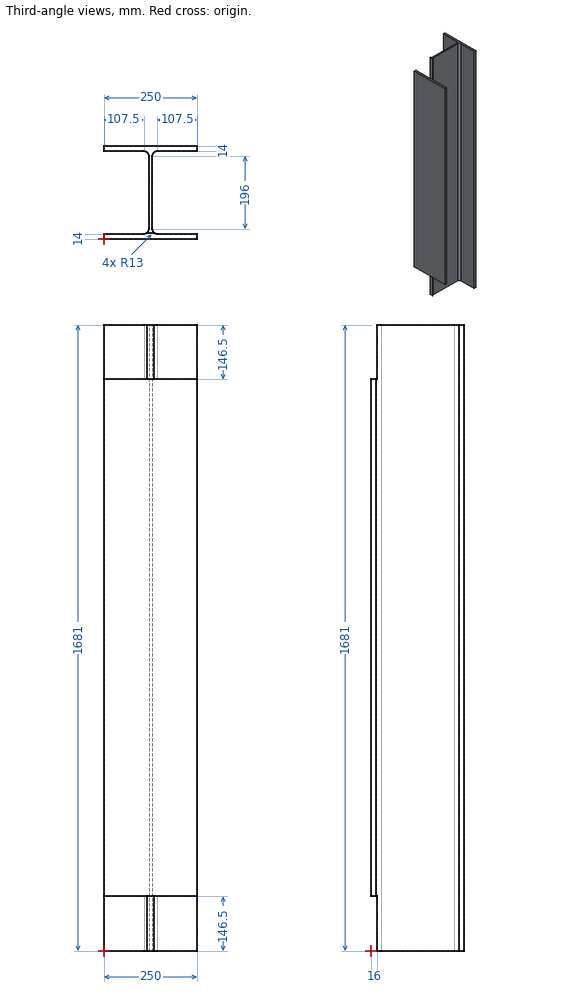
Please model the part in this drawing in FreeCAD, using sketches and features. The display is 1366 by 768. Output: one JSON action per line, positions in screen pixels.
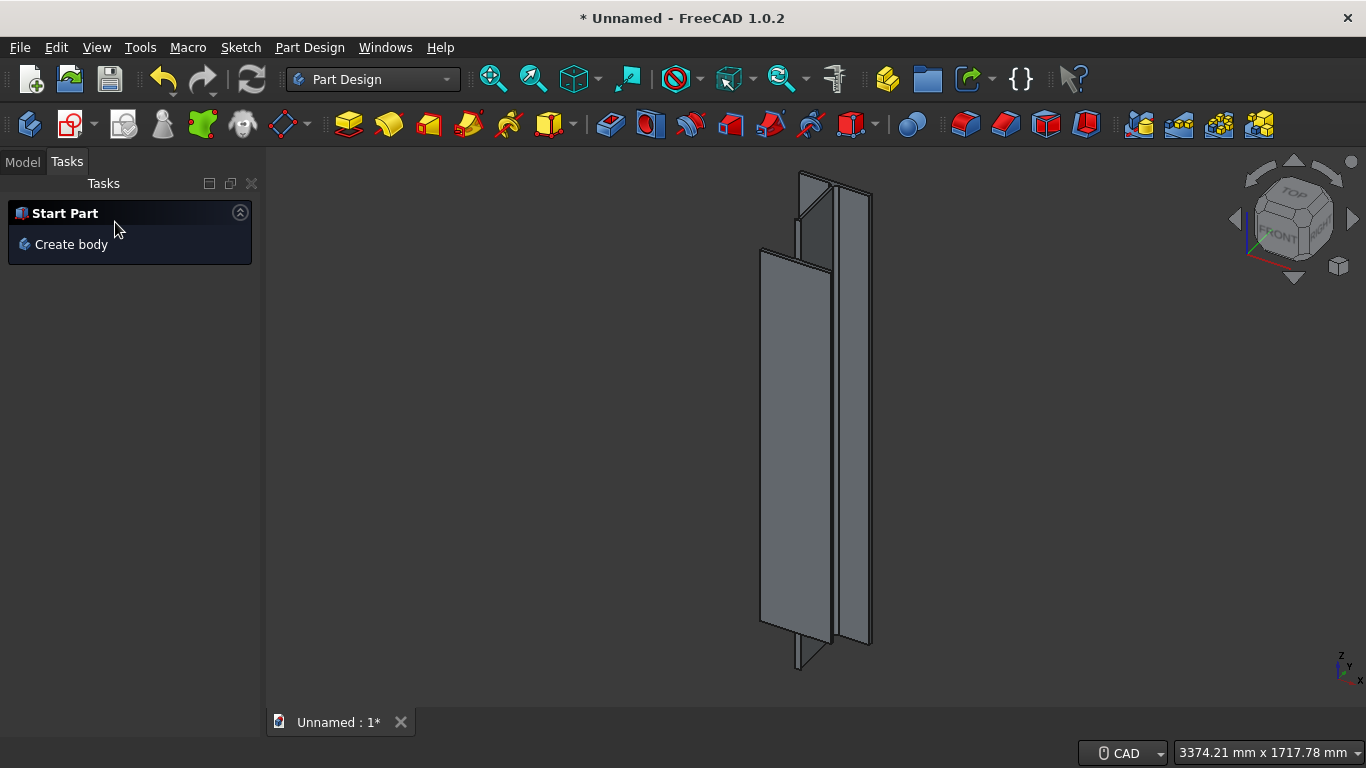
{"action": "key", "text": "0"}